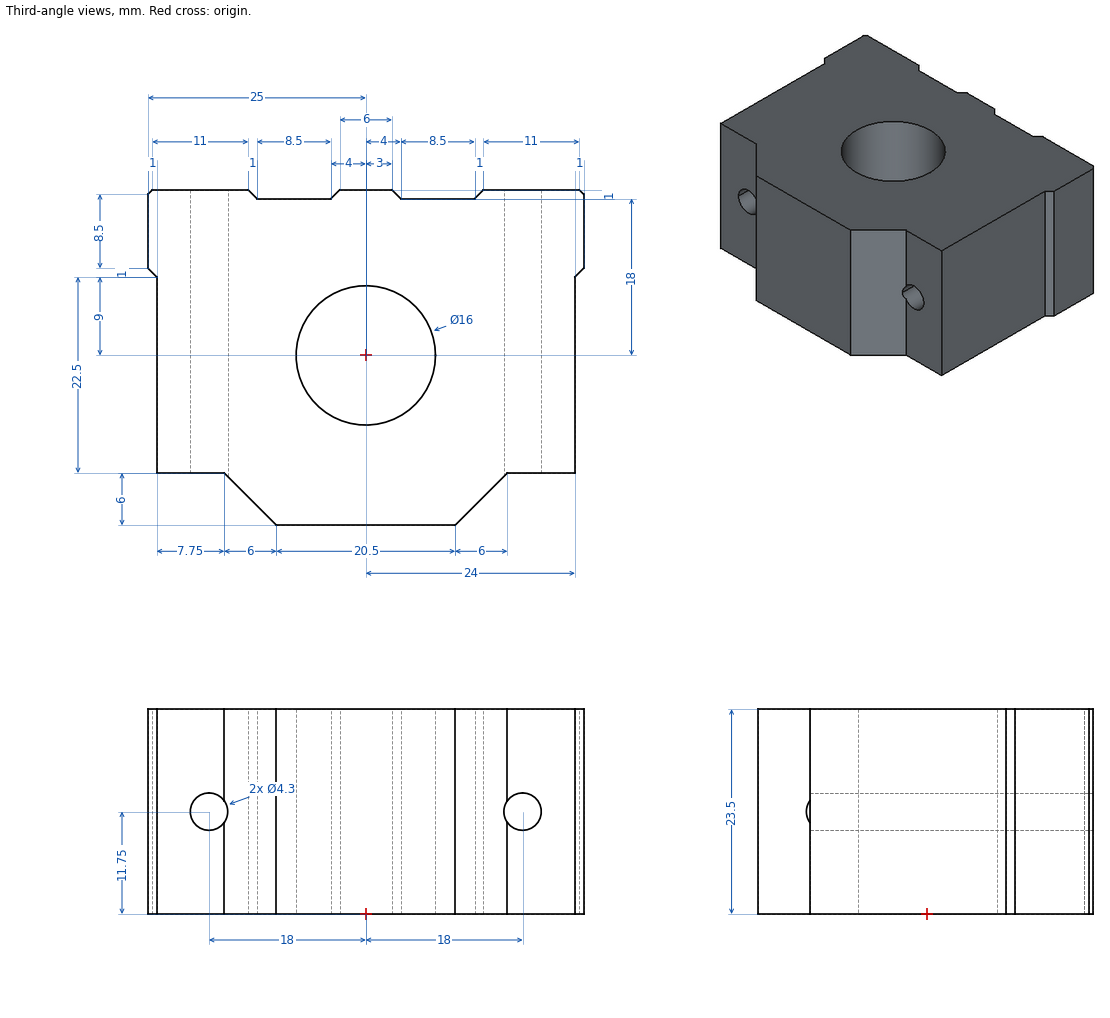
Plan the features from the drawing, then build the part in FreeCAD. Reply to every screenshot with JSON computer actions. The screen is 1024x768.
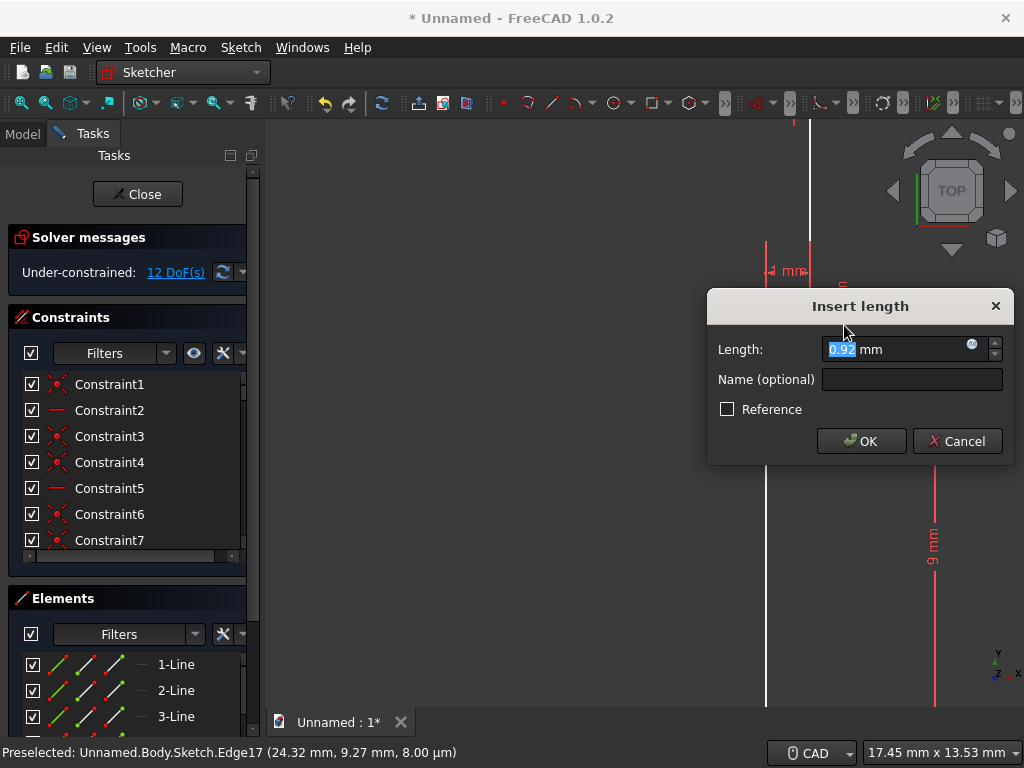
{"action": "type", "text": "1"}
{"action": "key", "text": "Return"}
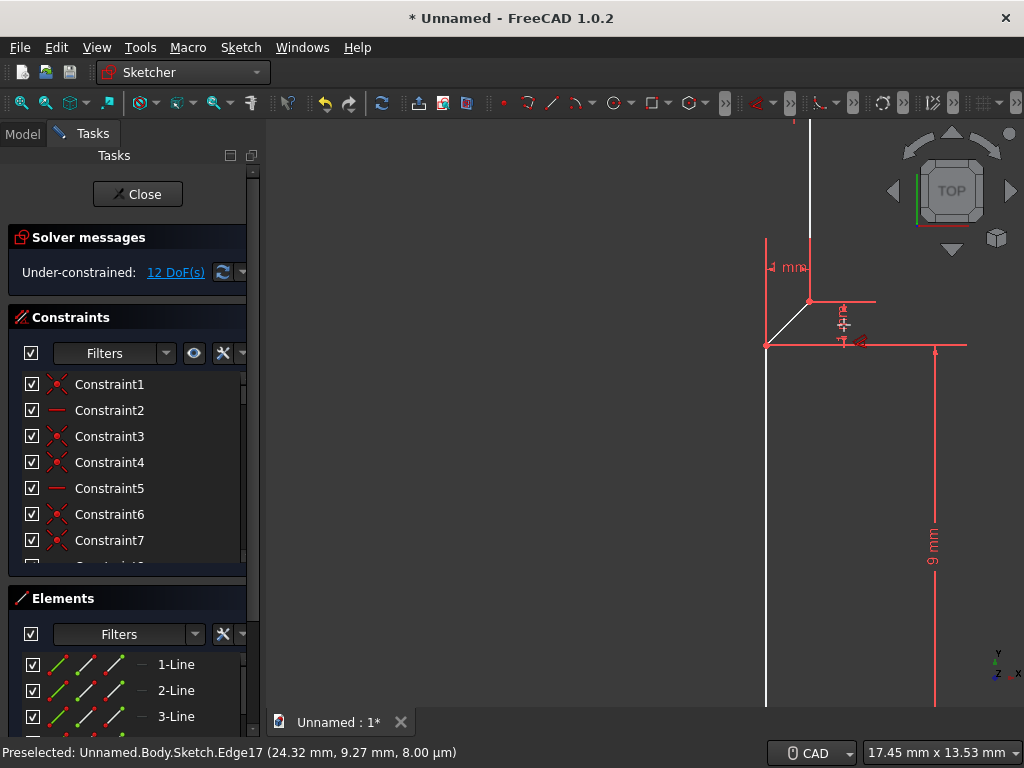
{"action": "scroll", "coordinate": [793, 328], "scroll_direction": "down", "scroll_amount": 8}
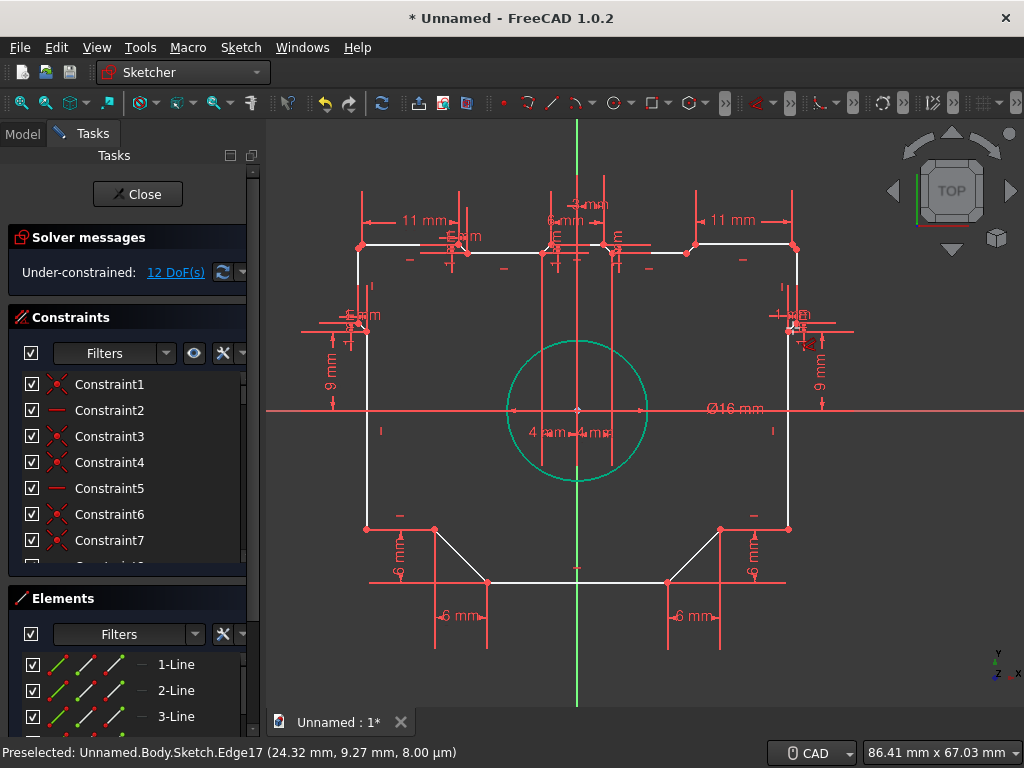
{"action": "scroll", "coordinate": [693, 247], "scroll_direction": "up", "scroll_amount": 8}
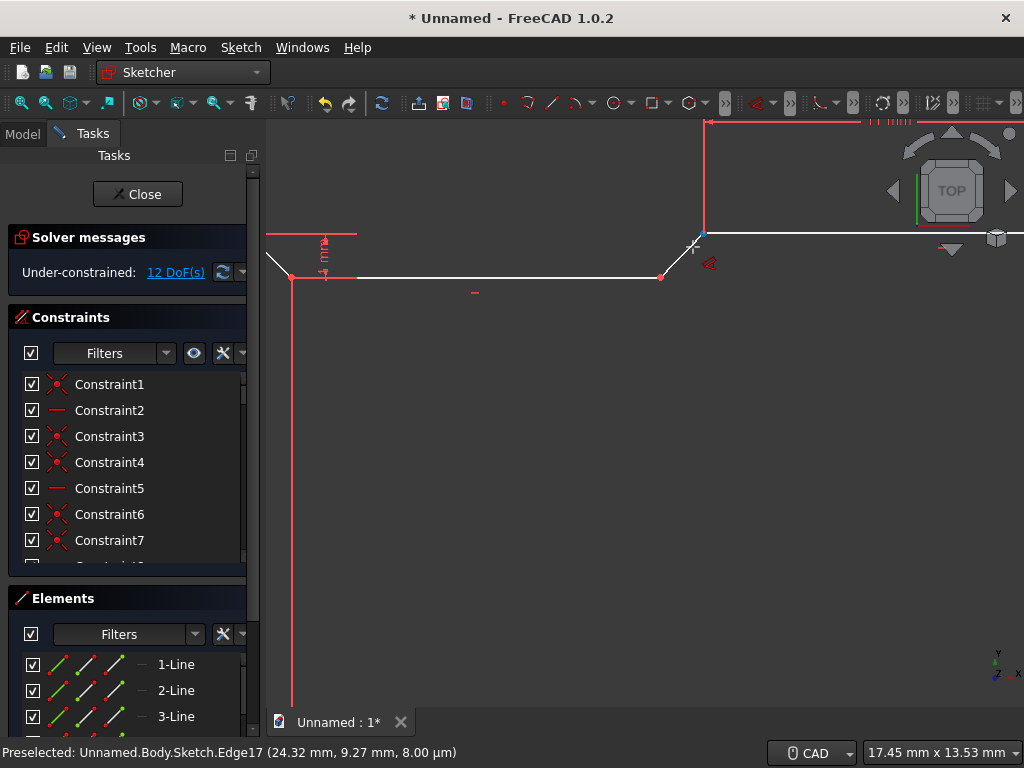
{"action": "left_click", "coordinate": [691, 247]}
{"action": "left_click", "coordinate": [682, 199]}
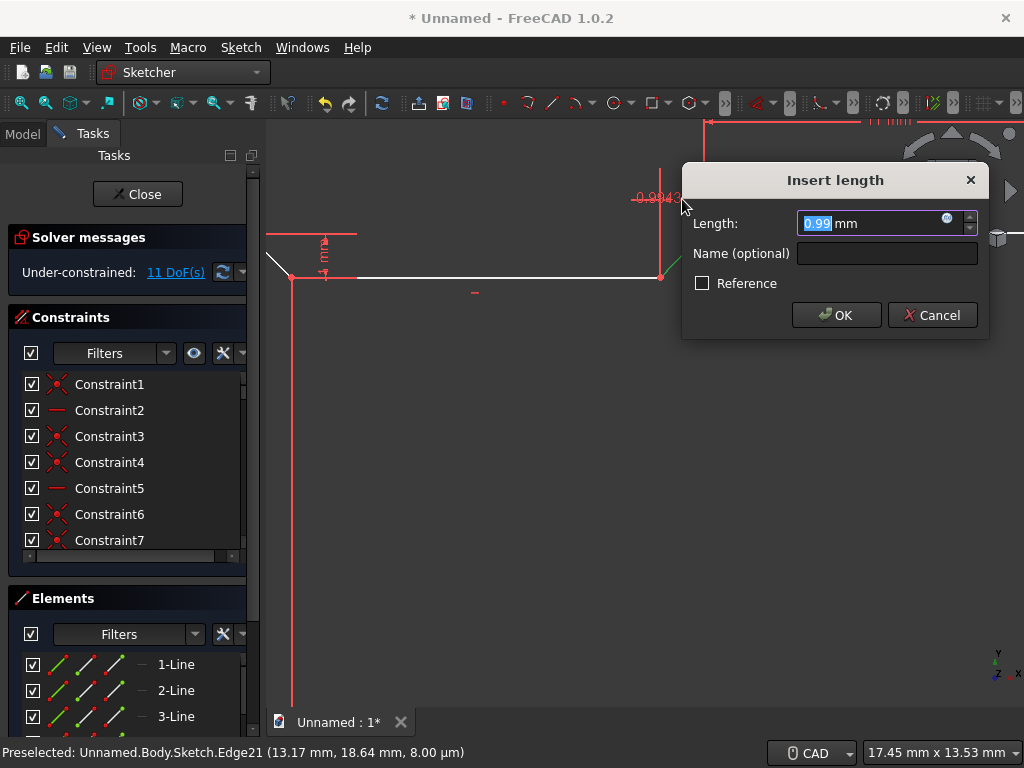
{"action": "type", "text": "1"}
{"action": "key", "text": "Return"}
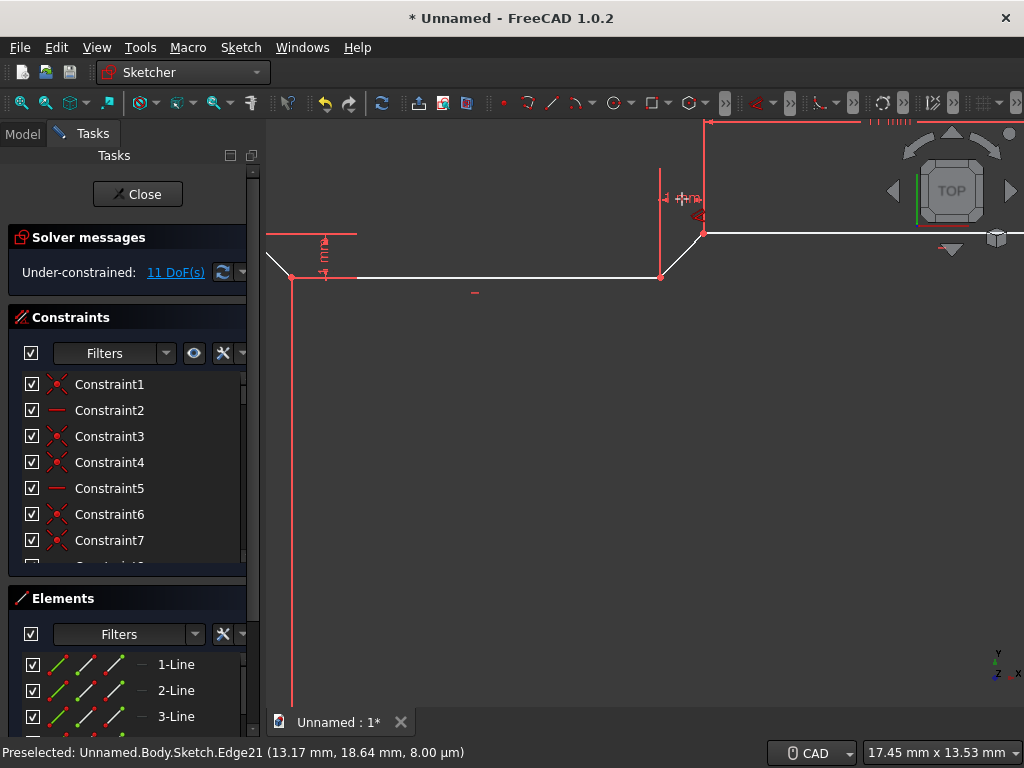
{"action": "left_click", "coordinate": [691, 247]}
{"action": "left_click", "coordinate": [738, 256]}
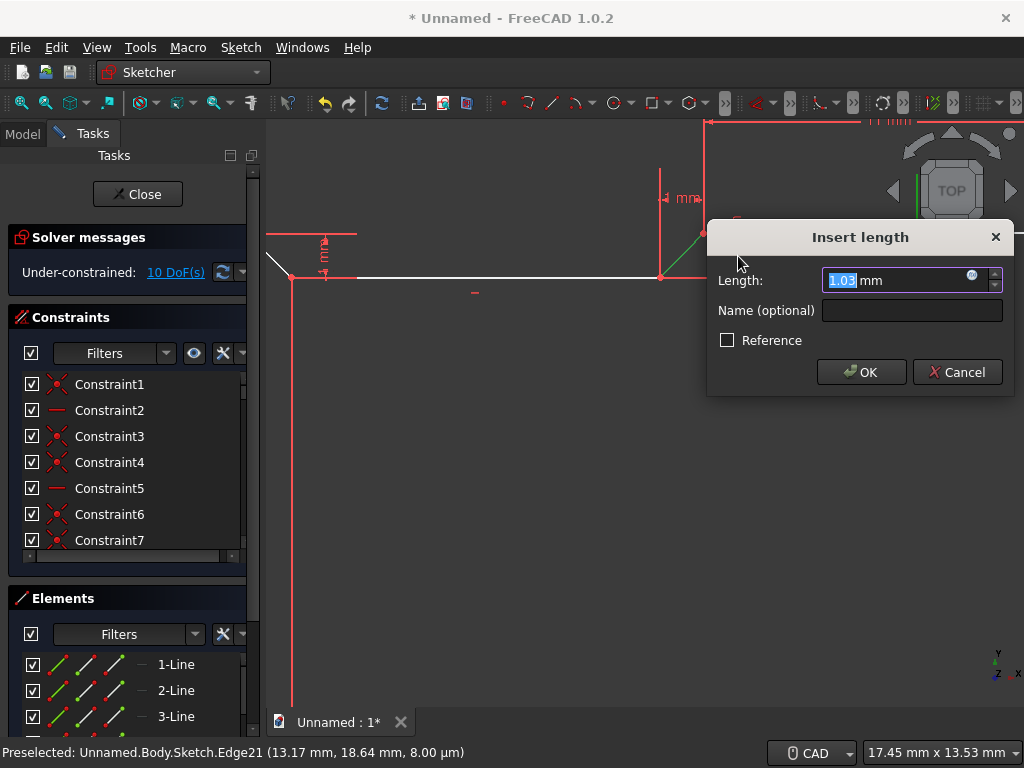
{"action": "type", "text": "1"}
{"action": "key", "text": "Return"}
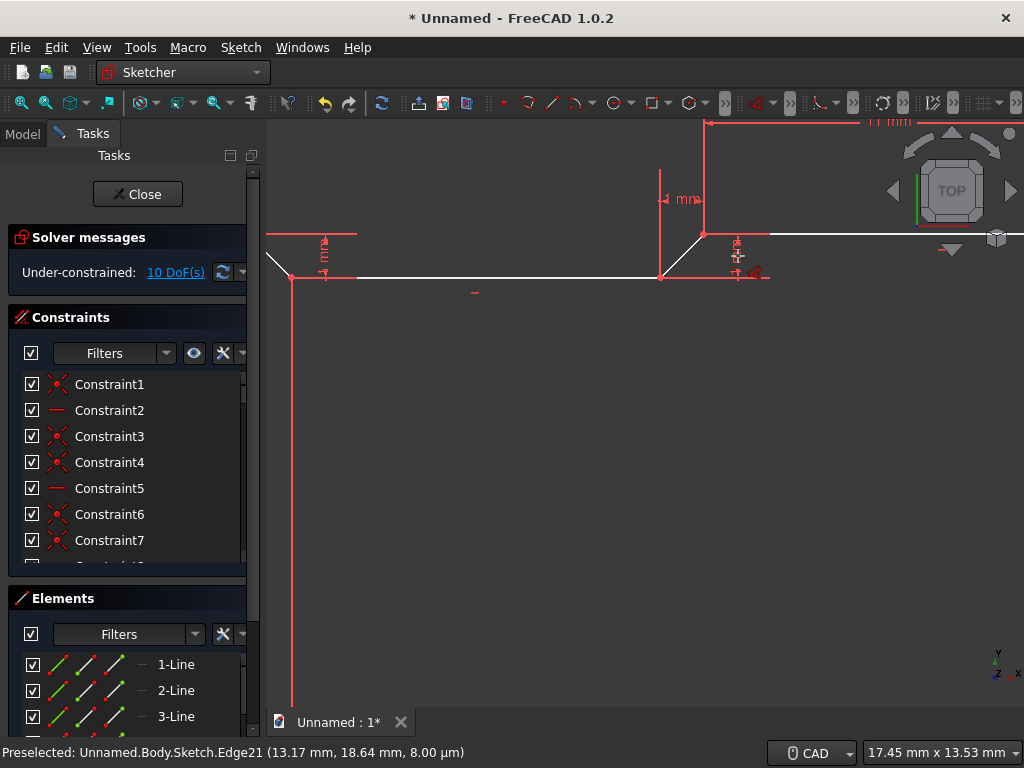
{"action": "scroll", "coordinate": [693, 247], "scroll_direction": "down", "scroll_amount": 8}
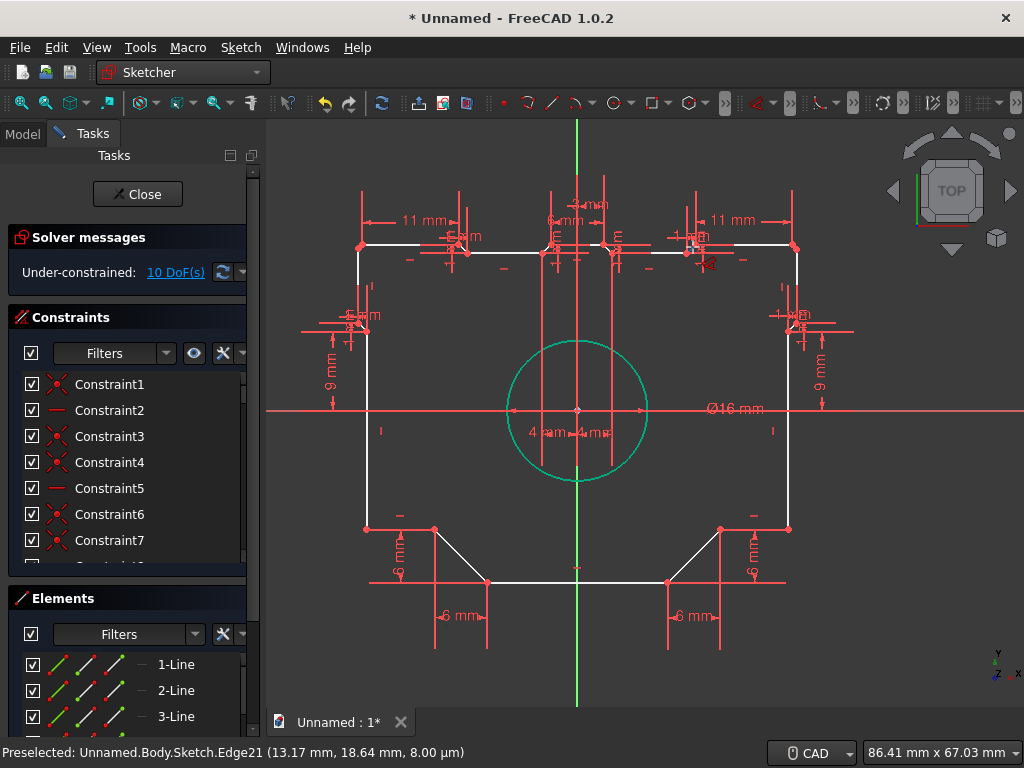
{"action": "left_click", "coordinate": [520, 253]}
{"action": "left_click", "coordinate": [505, 287]}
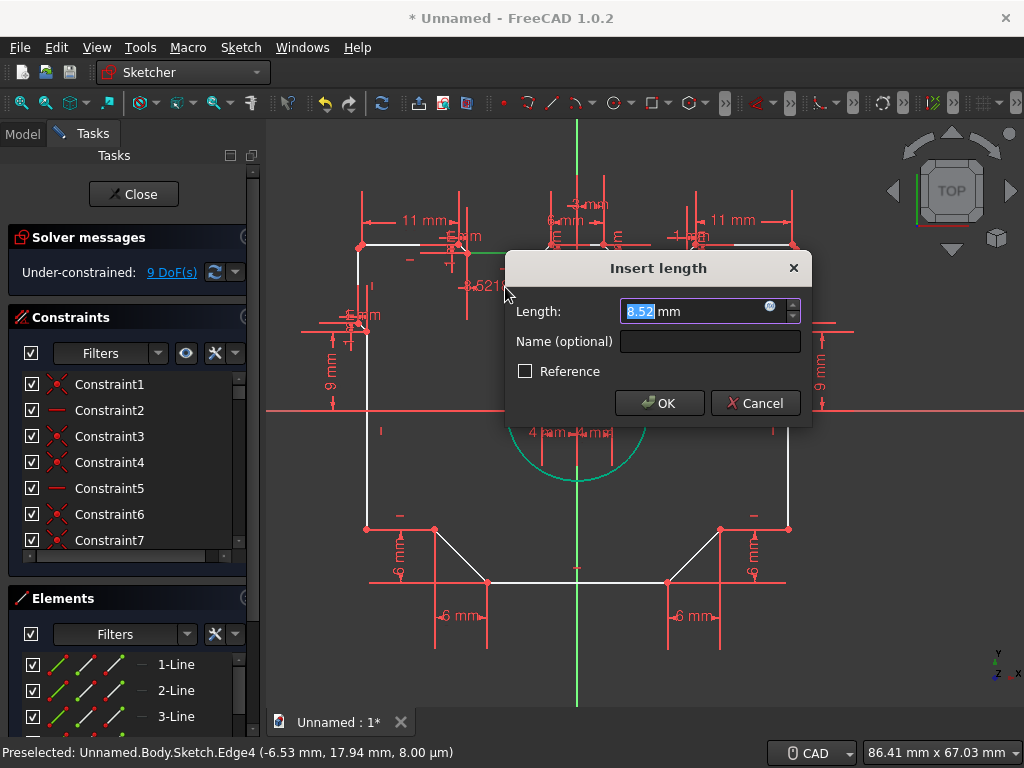
{"action": "type", "text": "8.5"}
{"action": "key", "text": "Return"}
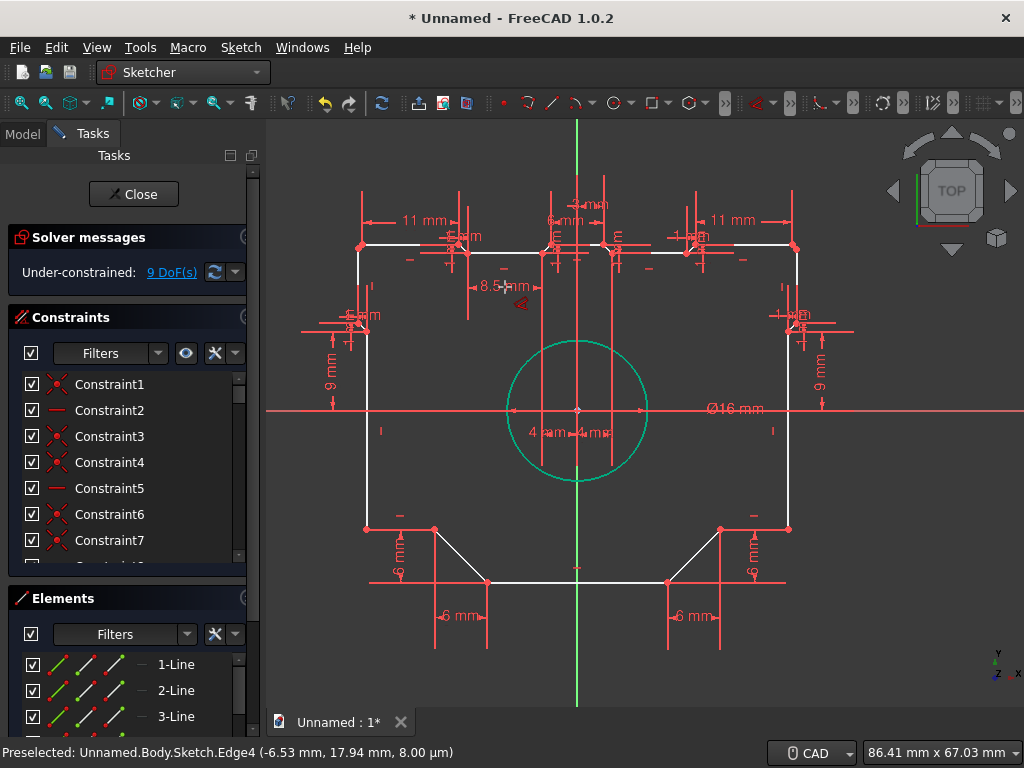
{"action": "left_click", "coordinate": [358, 271]}
{"action": "left_click", "coordinate": [324, 286]}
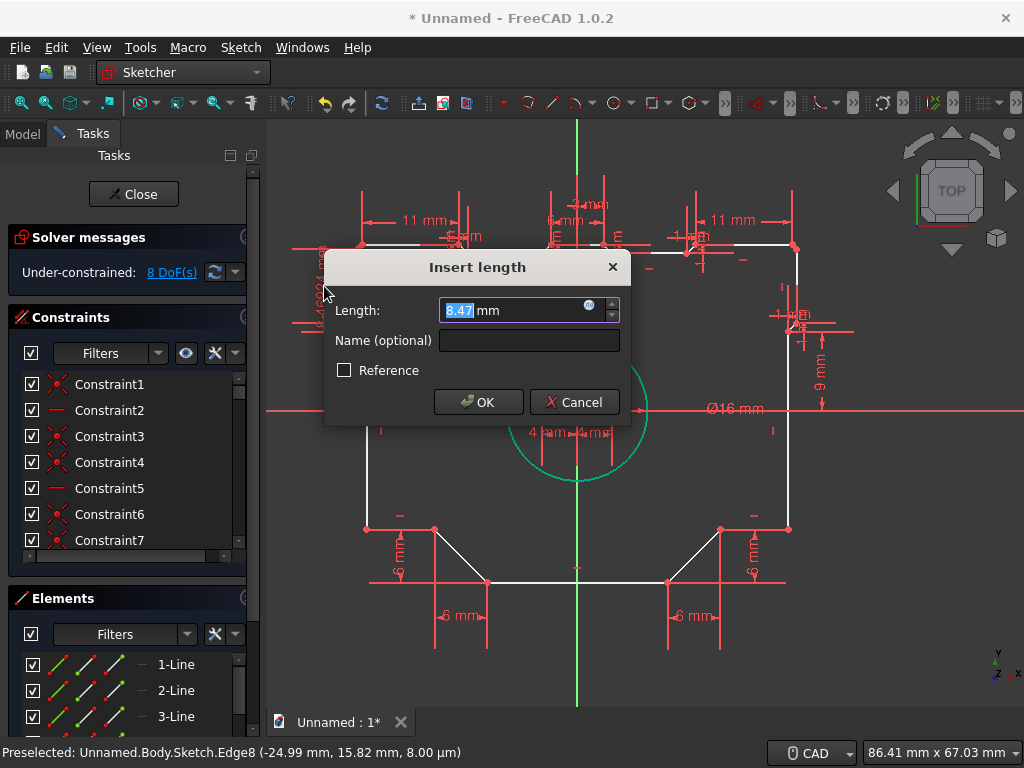
{"action": "type", "text": "8.5"}
{"action": "key", "text": "Return"}